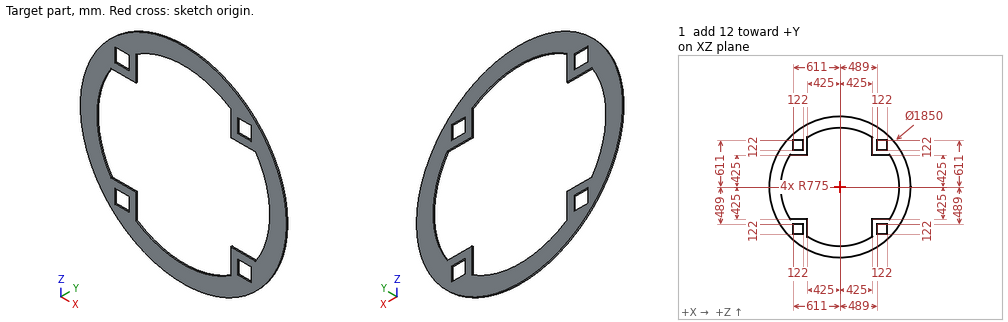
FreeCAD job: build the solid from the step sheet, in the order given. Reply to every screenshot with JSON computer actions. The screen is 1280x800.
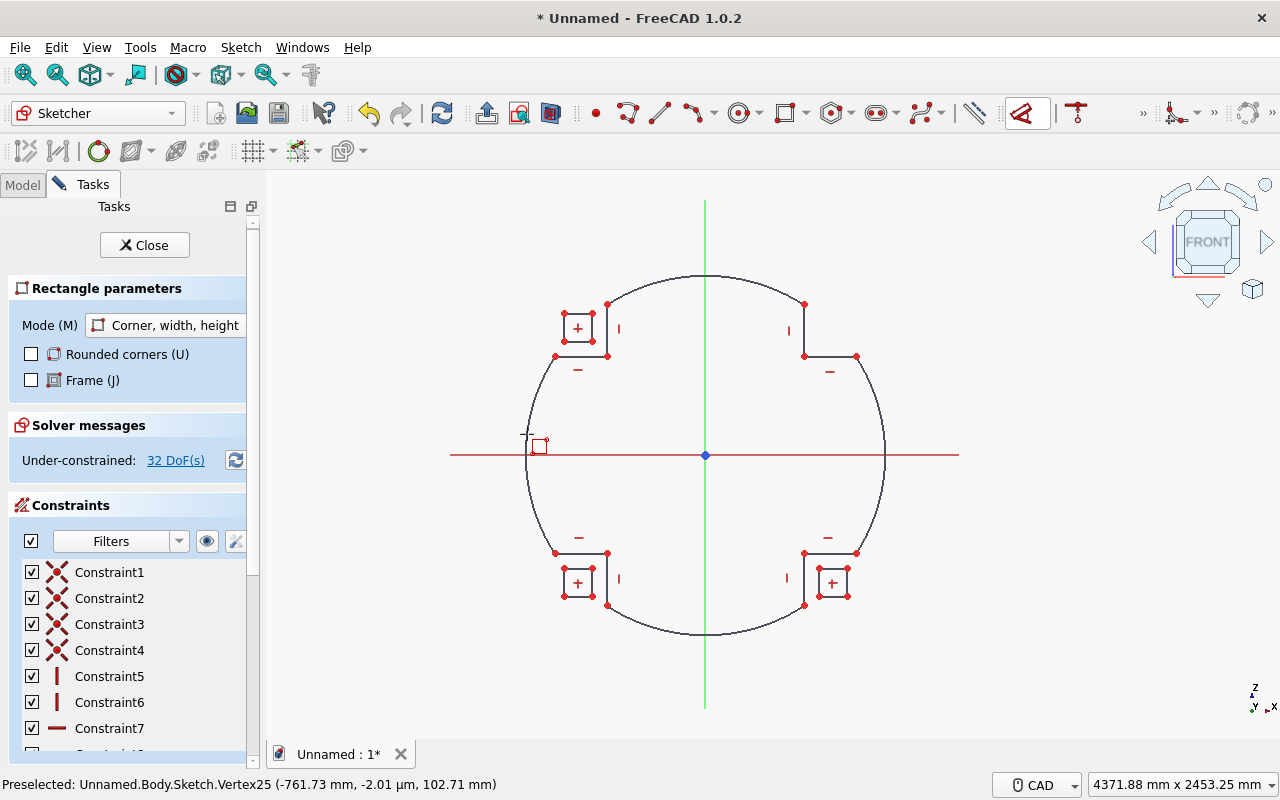
{"action": "left_click", "coordinate": [819, 313]}
{"action": "left_click", "coordinate": [847, 341]}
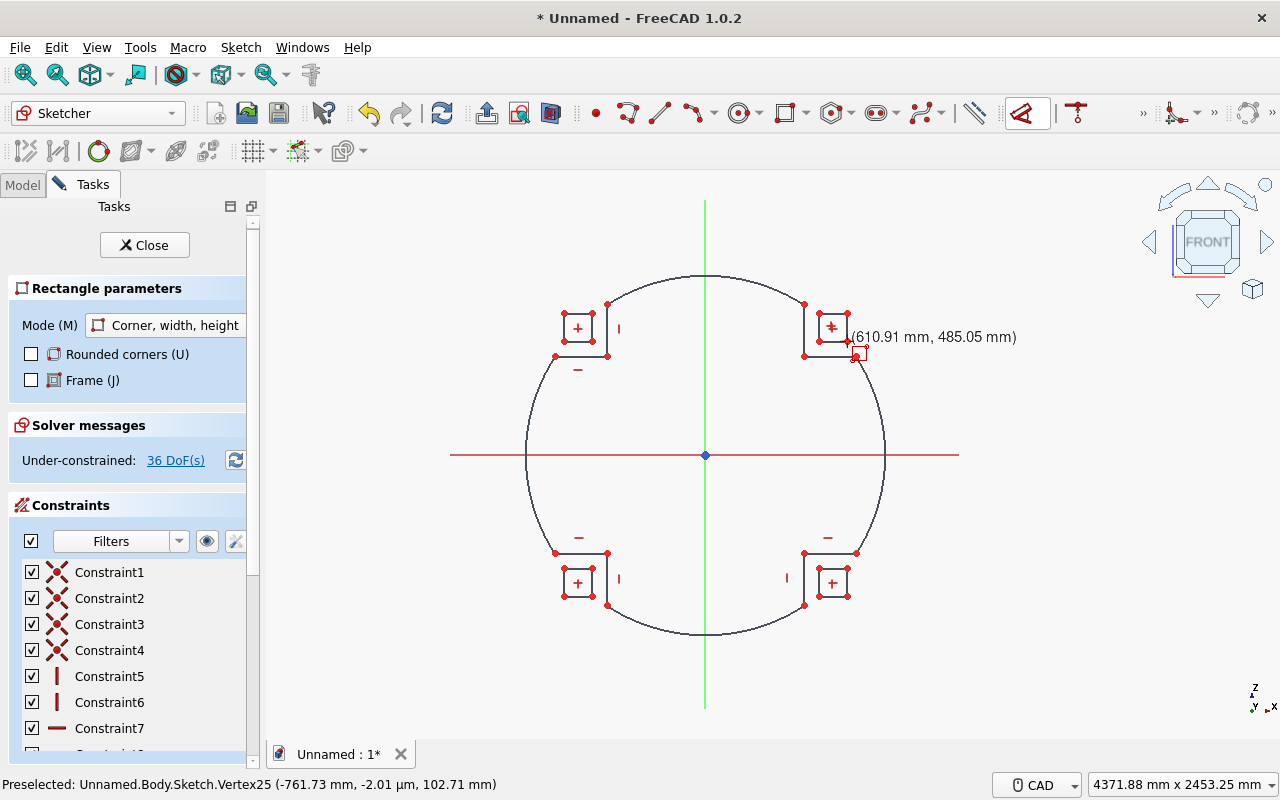
{"action": "key", "text": "g c"}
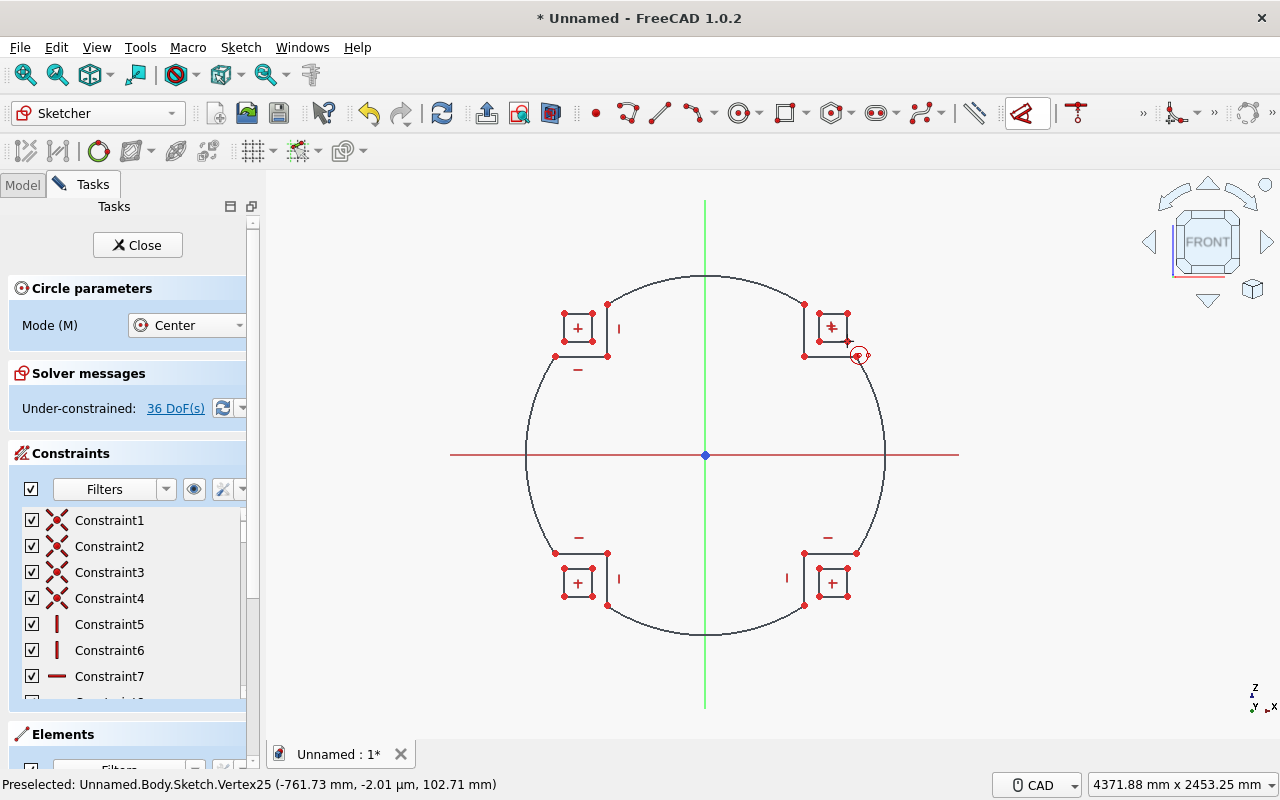
{"action": "left_click", "coordinate": [705, 454]}
{"action": "left_click", "coordinate": [857, 303]}
{"action": "key", "text": "Escape"}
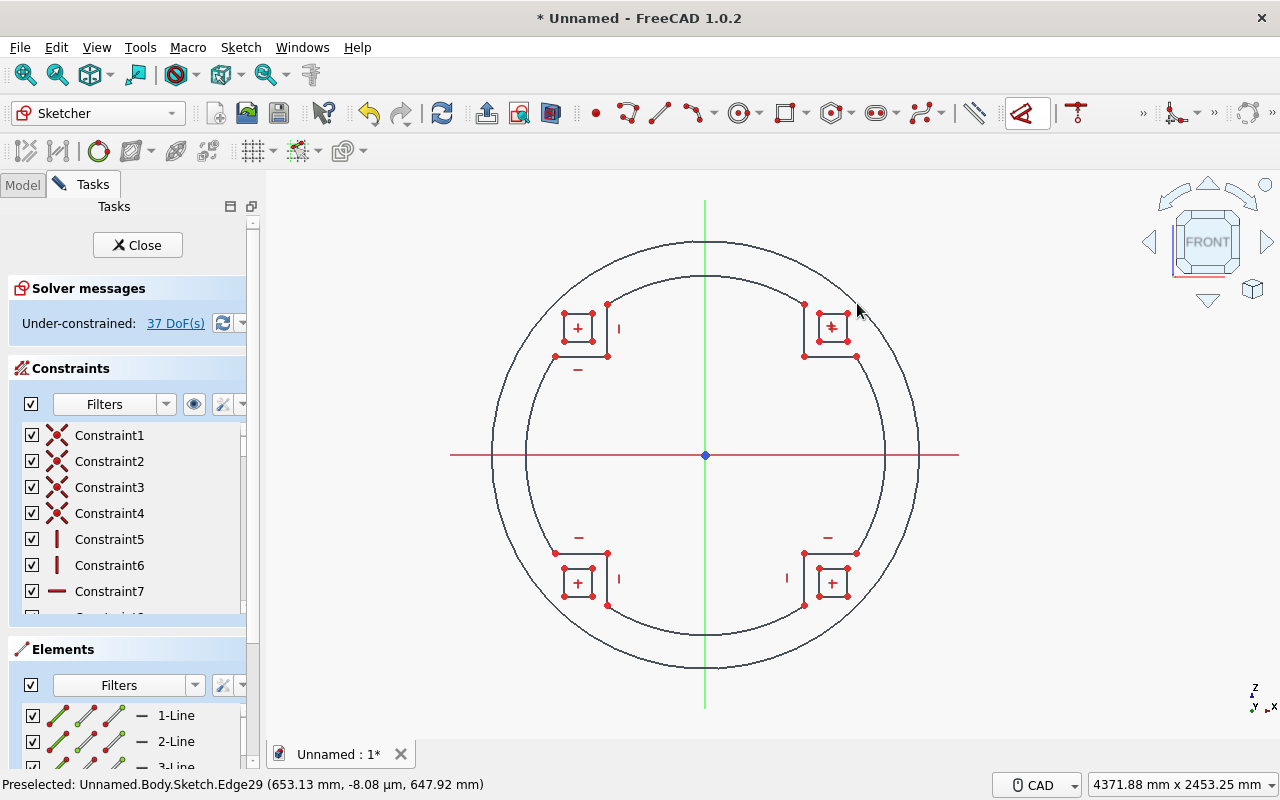
{"action": "left_click", "coordinate": [856, 303]}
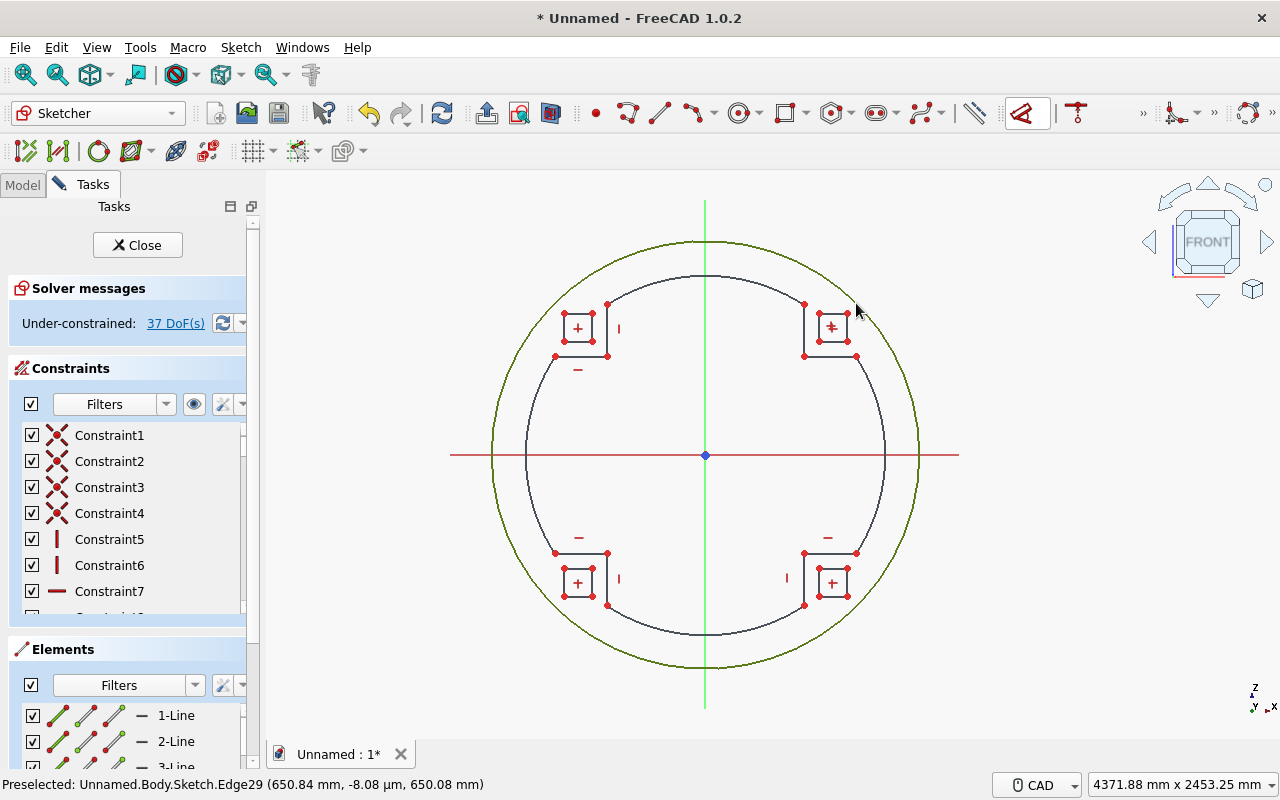
{"action": "left_click", "coordinate": [880, 497]}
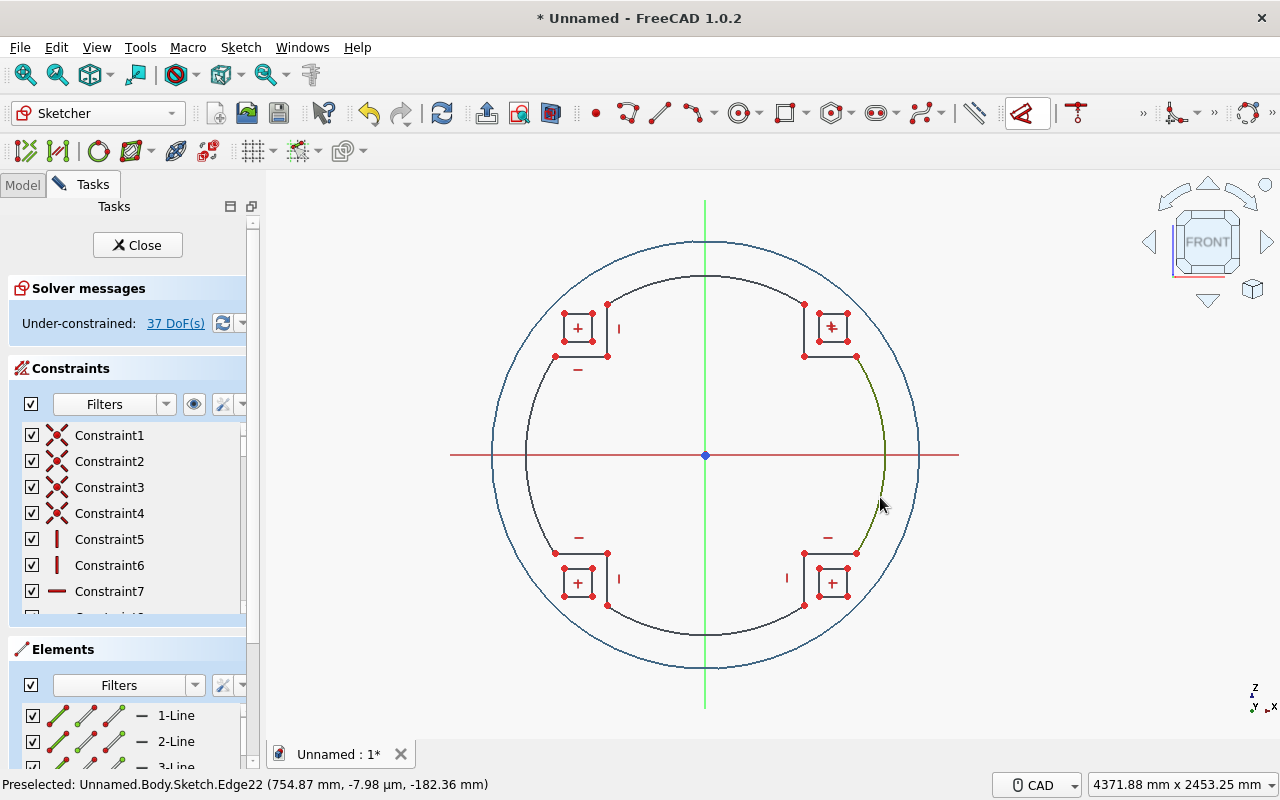
{"action": "left_click", "coordinate": [1076, 114]}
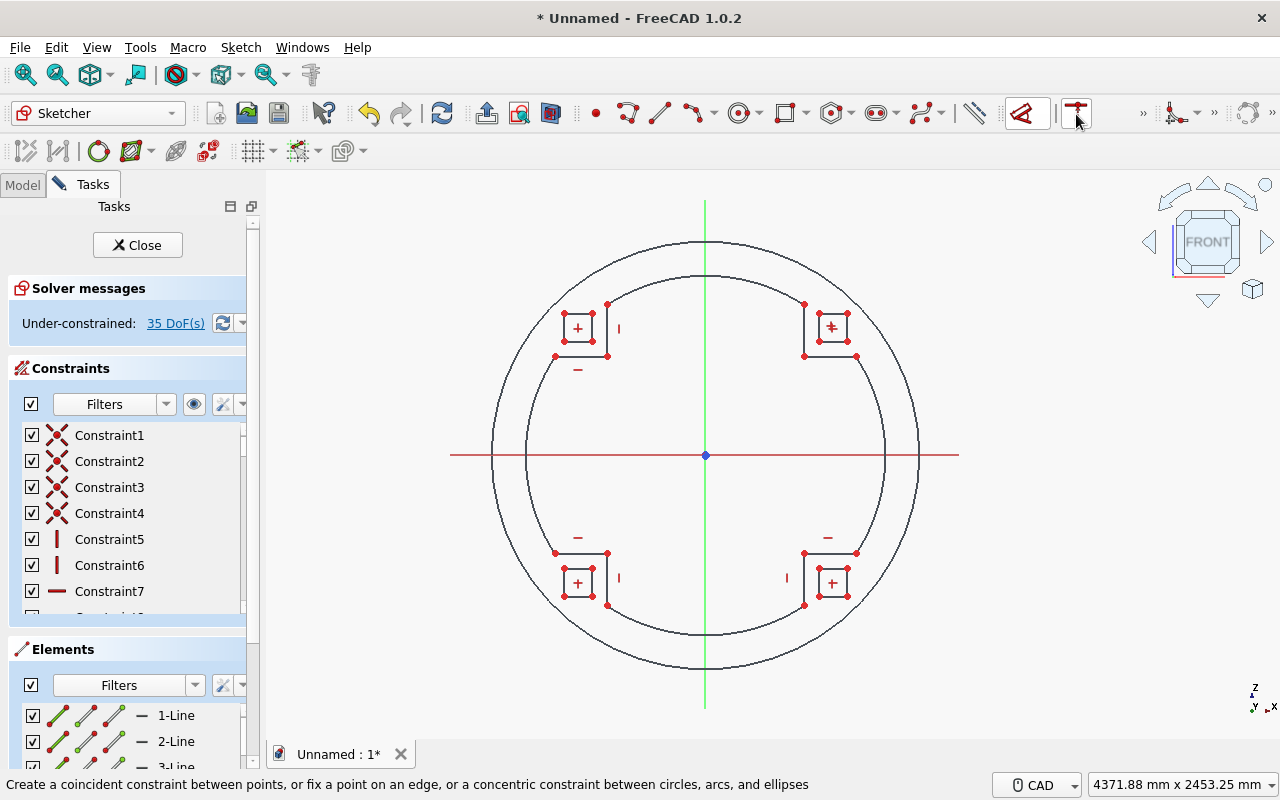
{"action": "left_click", "coordinate": [856, 304]}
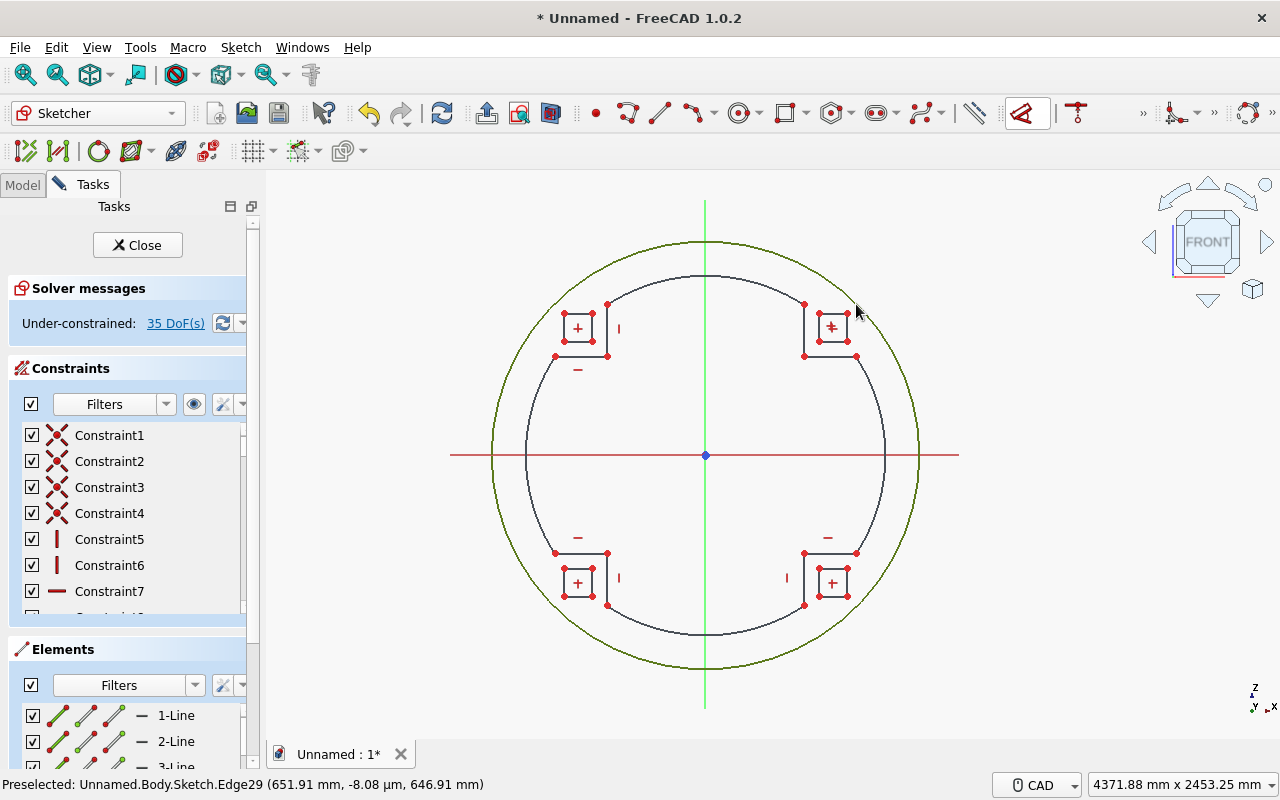
{"action": "left_click", "coordinate": [747, 281]}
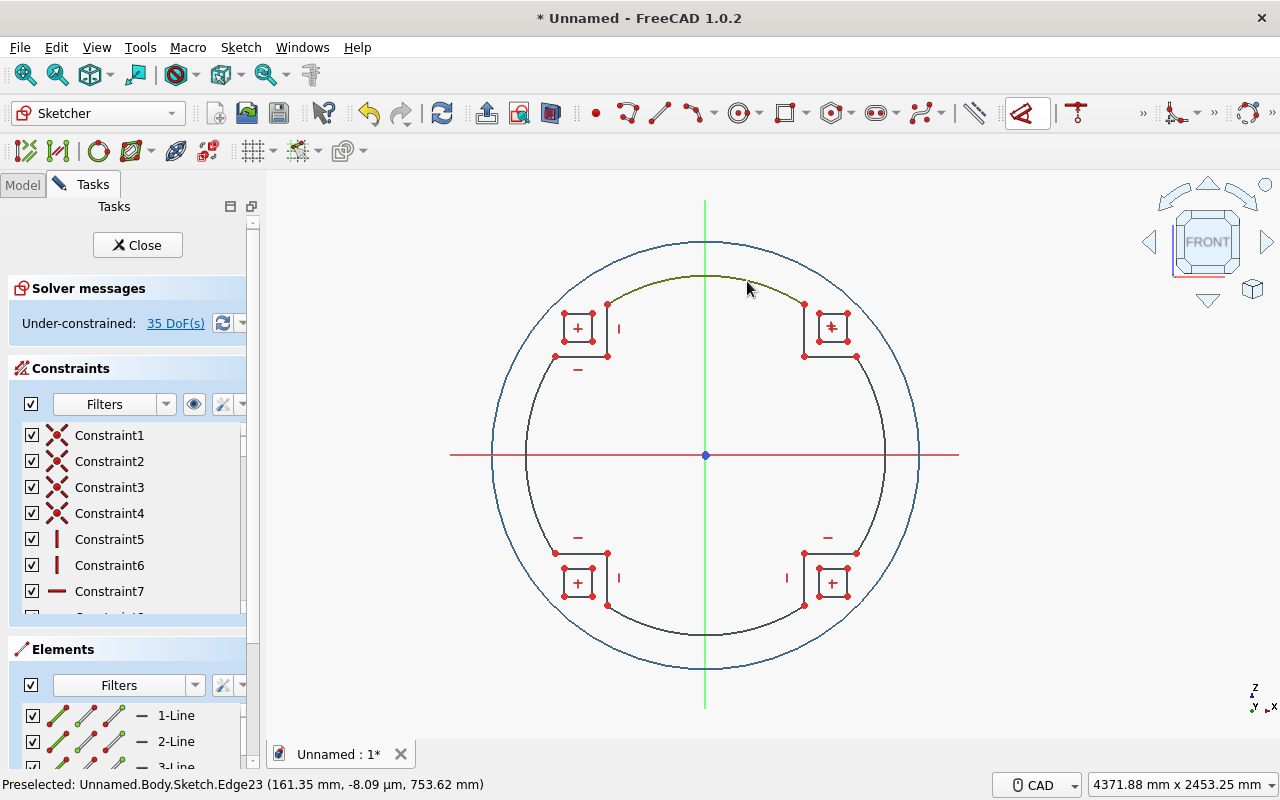
{"action": "key", "text": "c"}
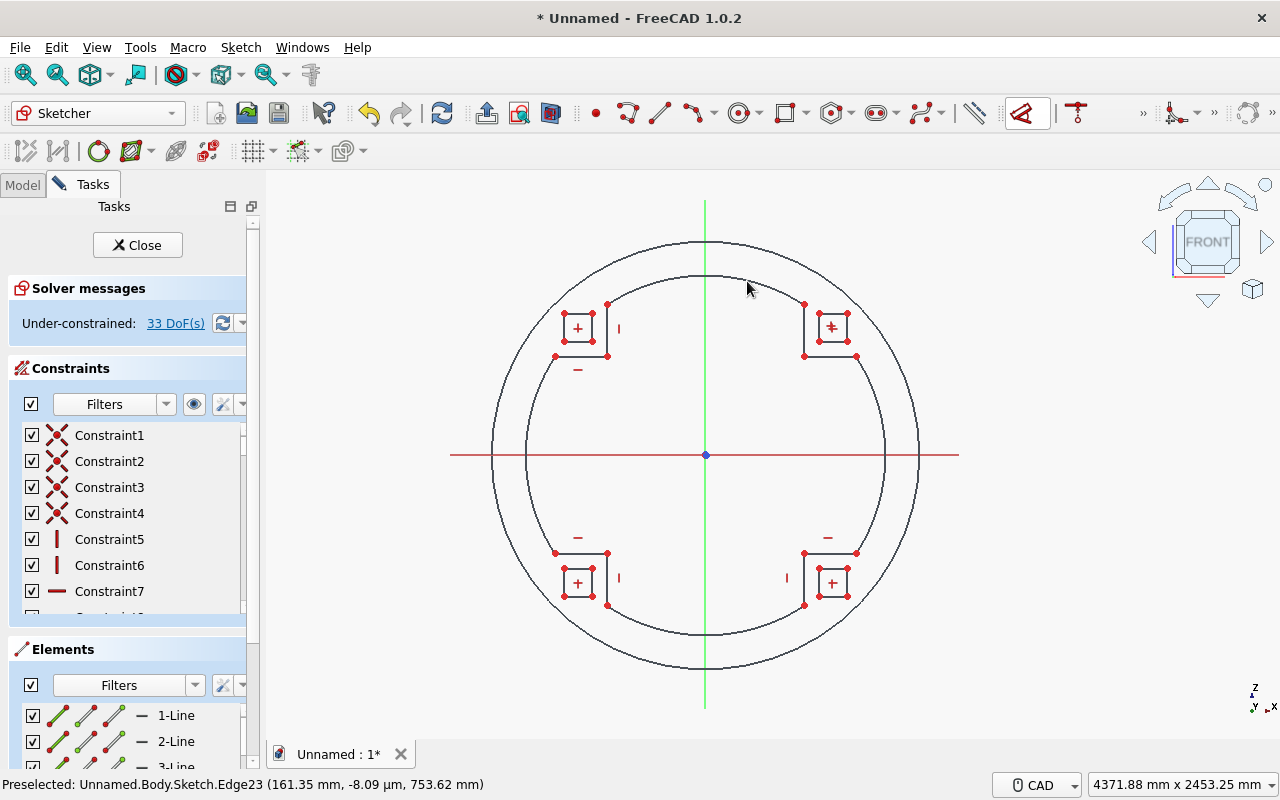
{"action": "left_click", "coordinate": [856, 304]}